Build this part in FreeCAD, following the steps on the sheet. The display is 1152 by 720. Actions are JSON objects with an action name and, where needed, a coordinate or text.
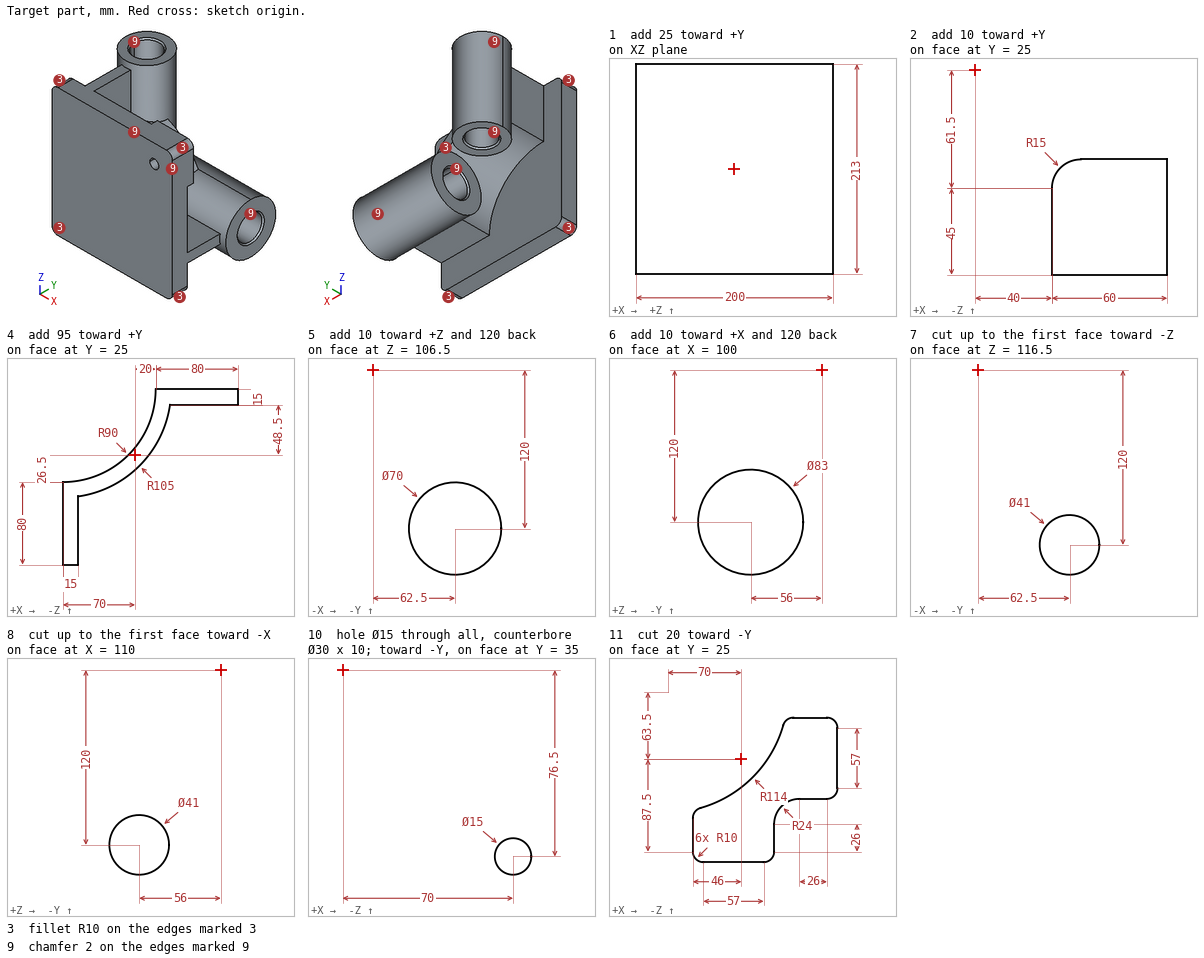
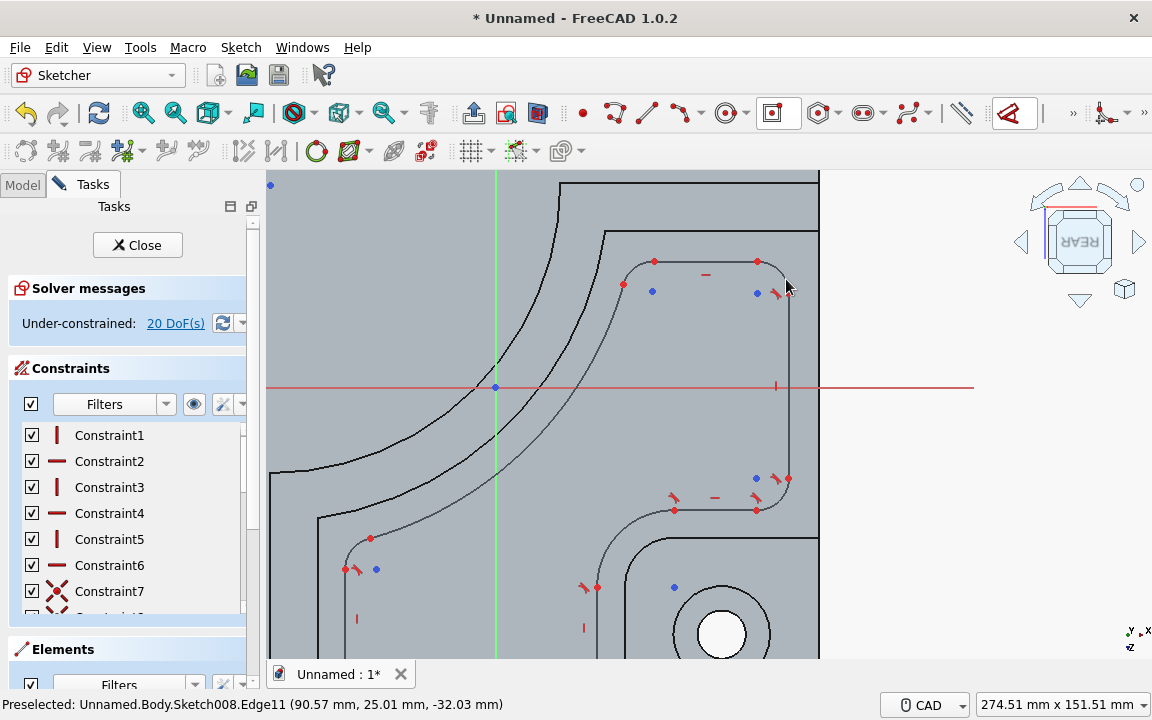
{"action": "left_click", "coordinate": [727, 262]}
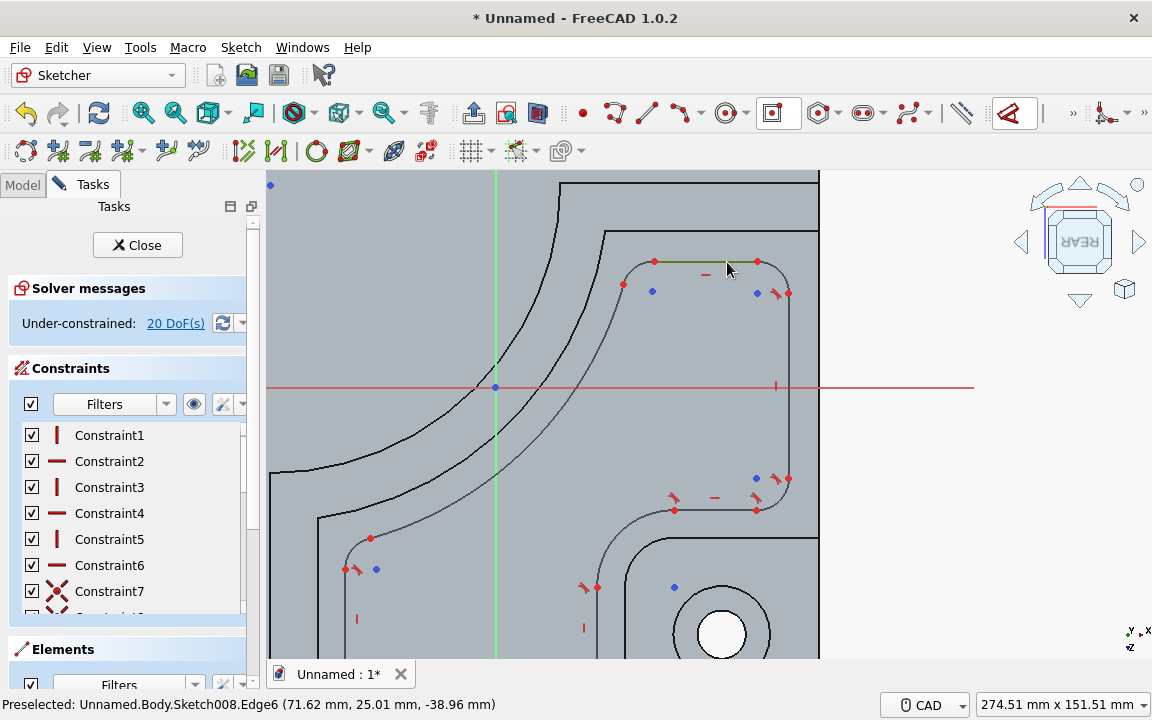
{"action": "left_click", "coordinate": [786, 279]}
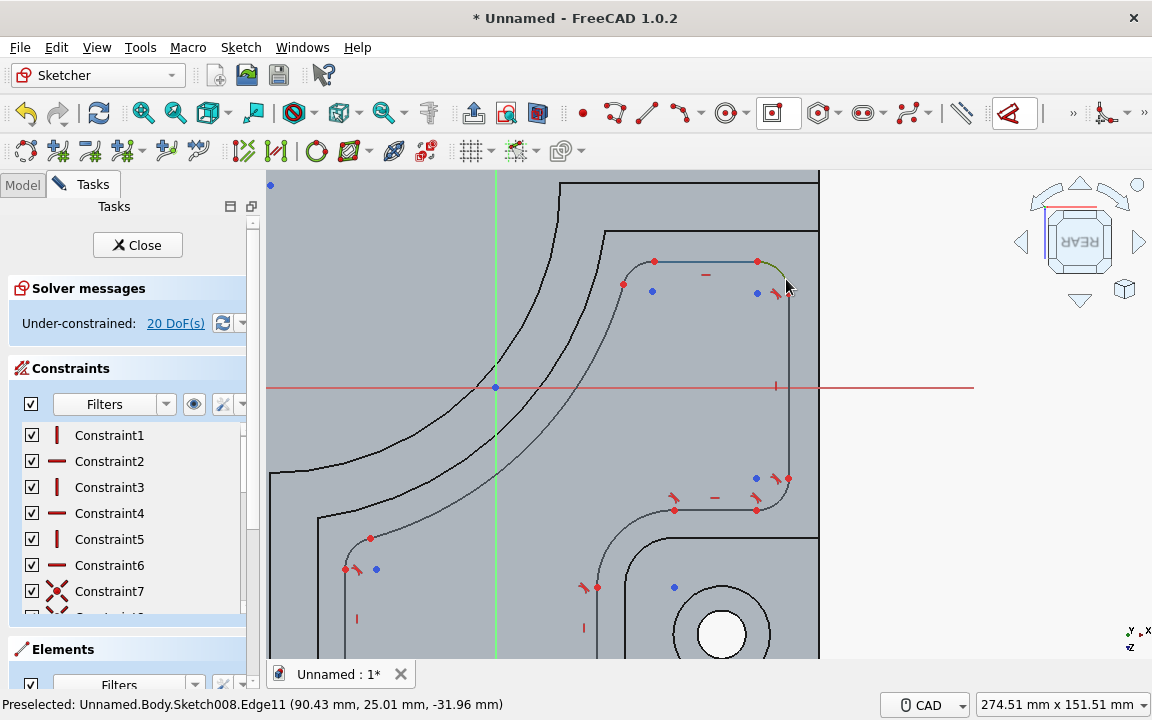
{"action": "key", "text": "t"}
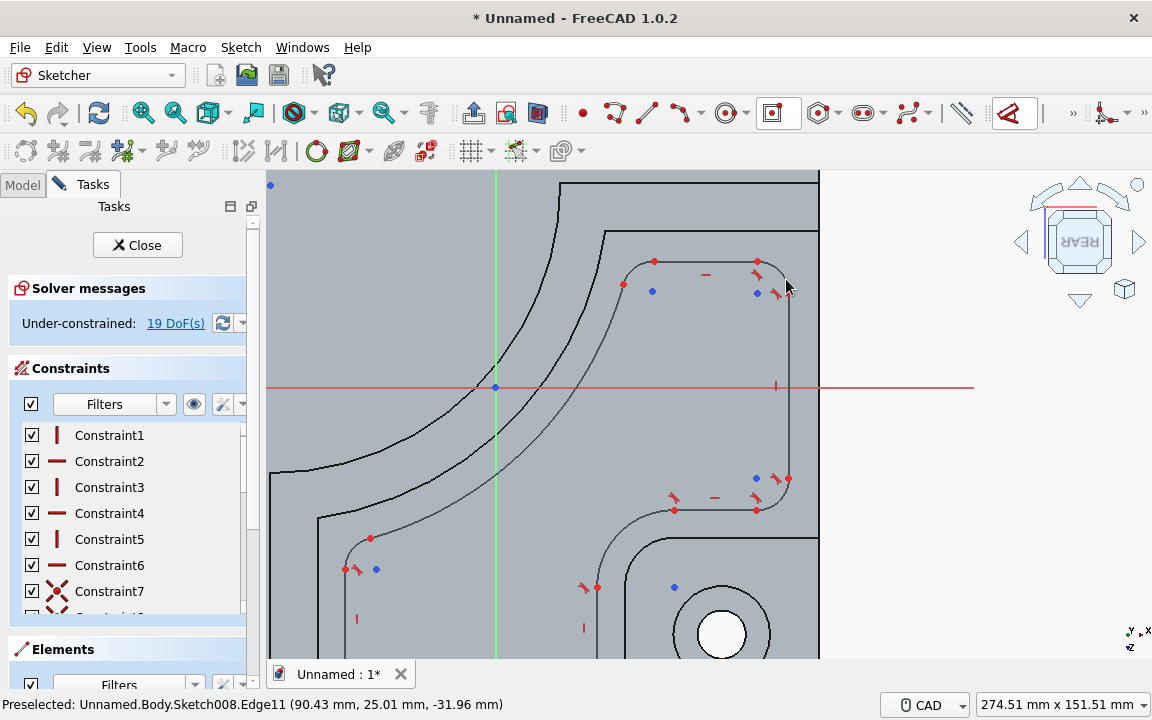
{"action": "left_click", "coordinate": [727, 262]}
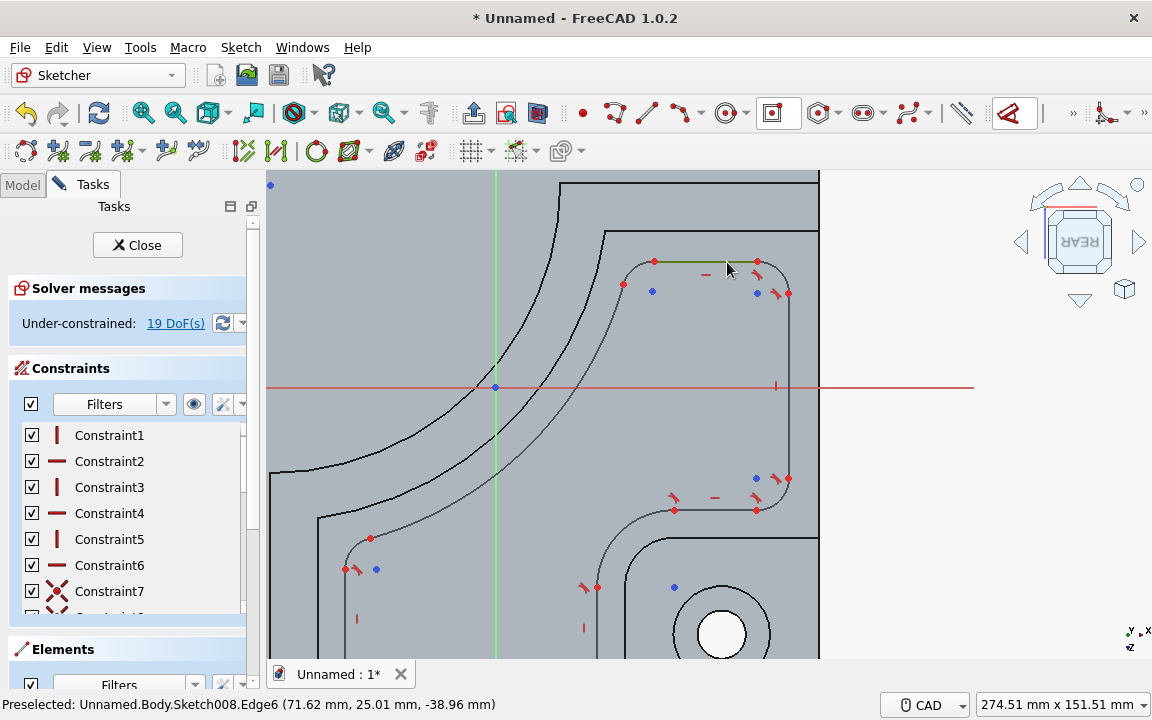
{"action": "left_click", "coordinate": [642, 264]}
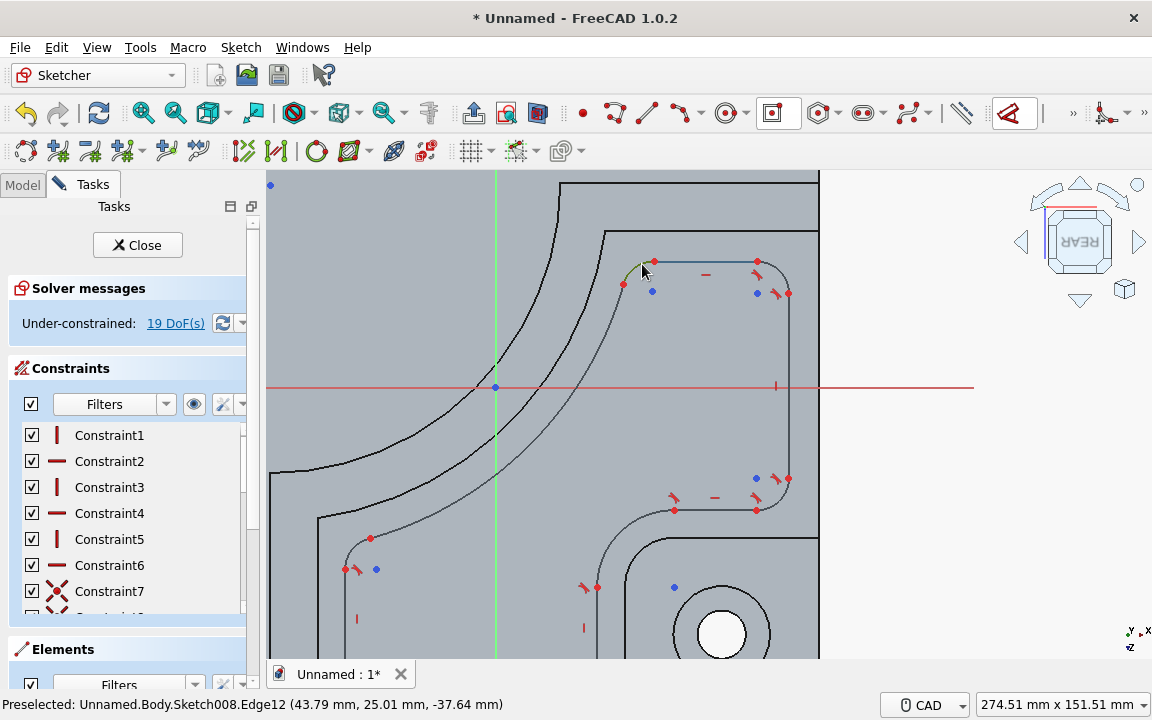
{"action": "key", "text": "t"}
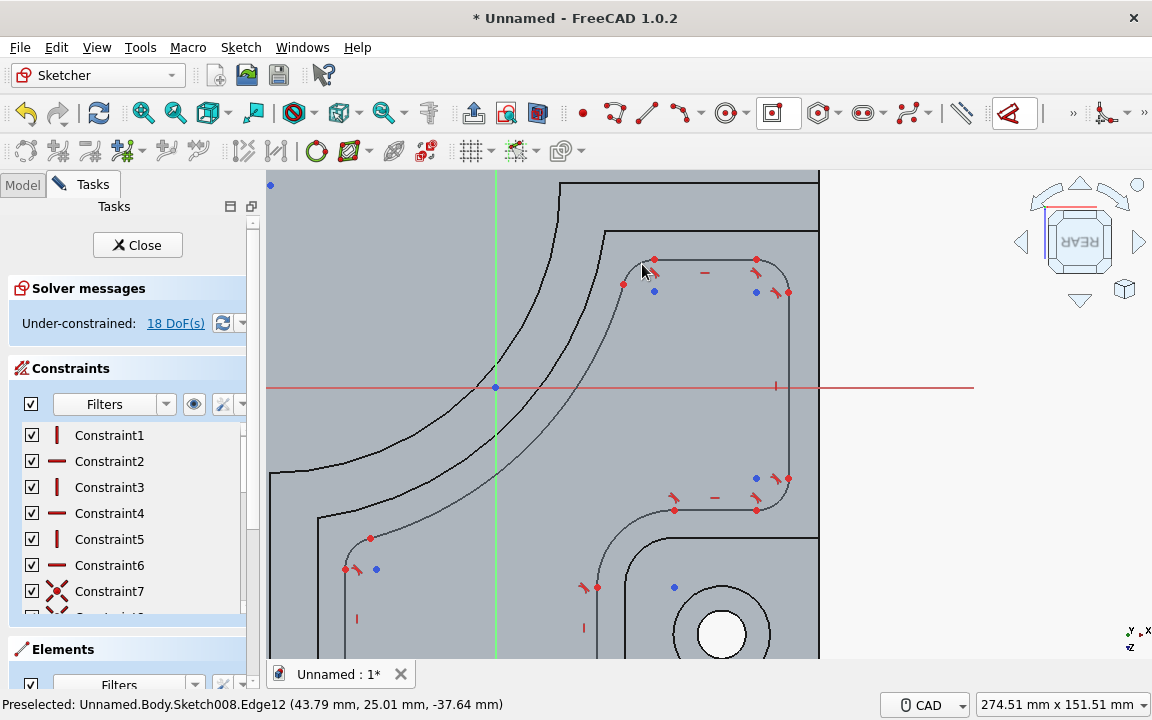
{"action": "left_click", "coordinate": [642, 262]}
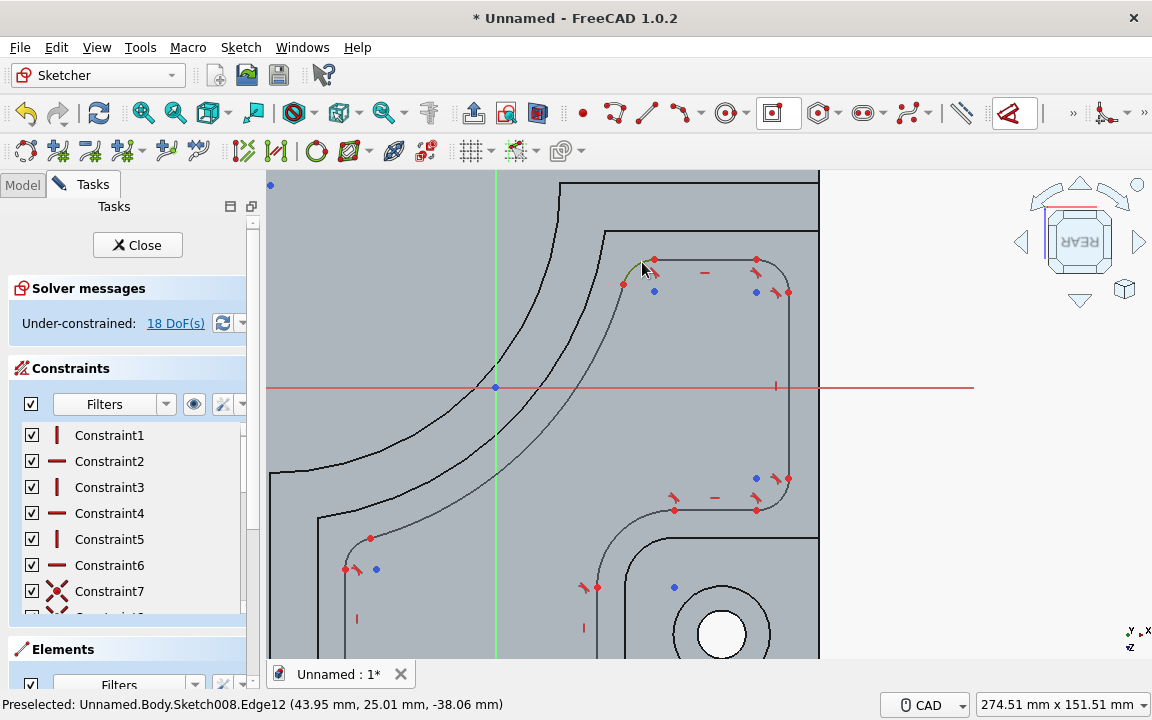
{"action": "left_click", "coordinate": [472, 492]}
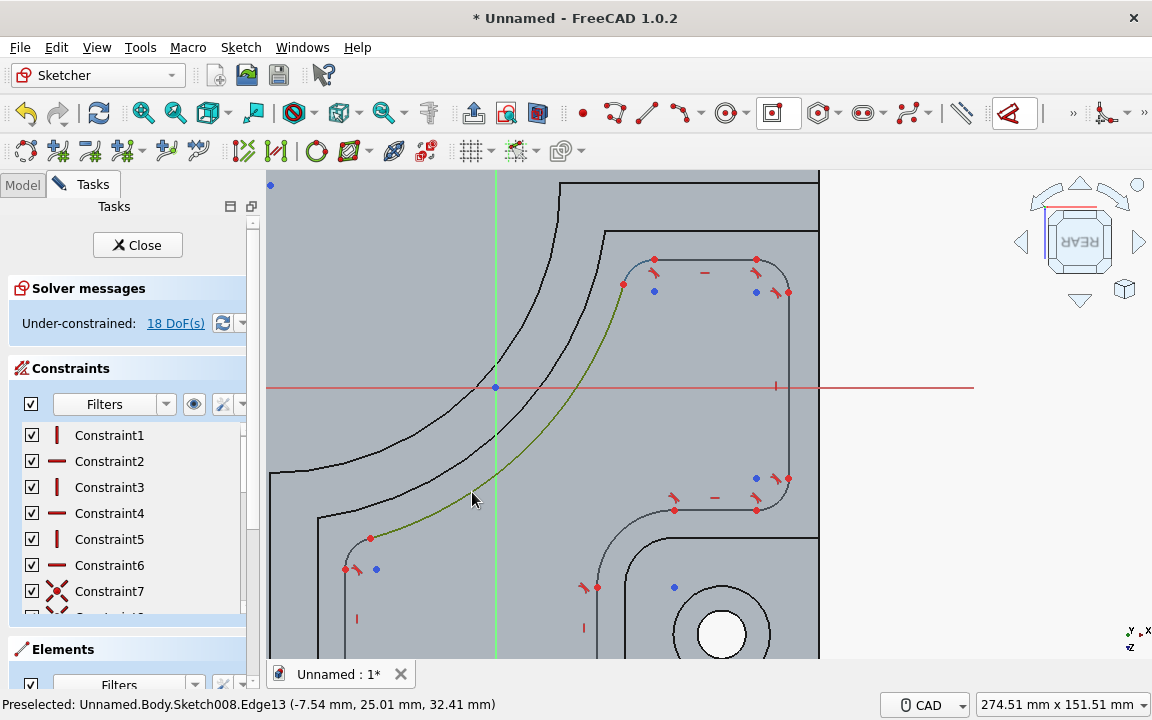
{"action": "key", "text": "t"}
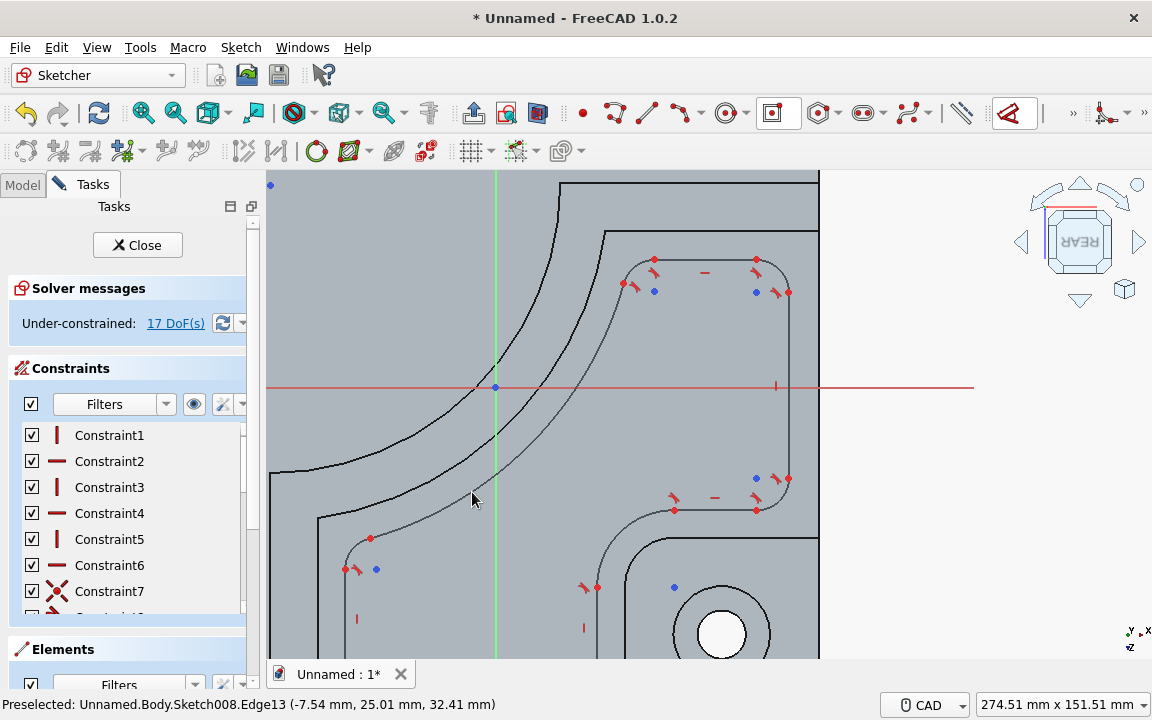
{"action": "left_click", "coordinate": [473, 492]}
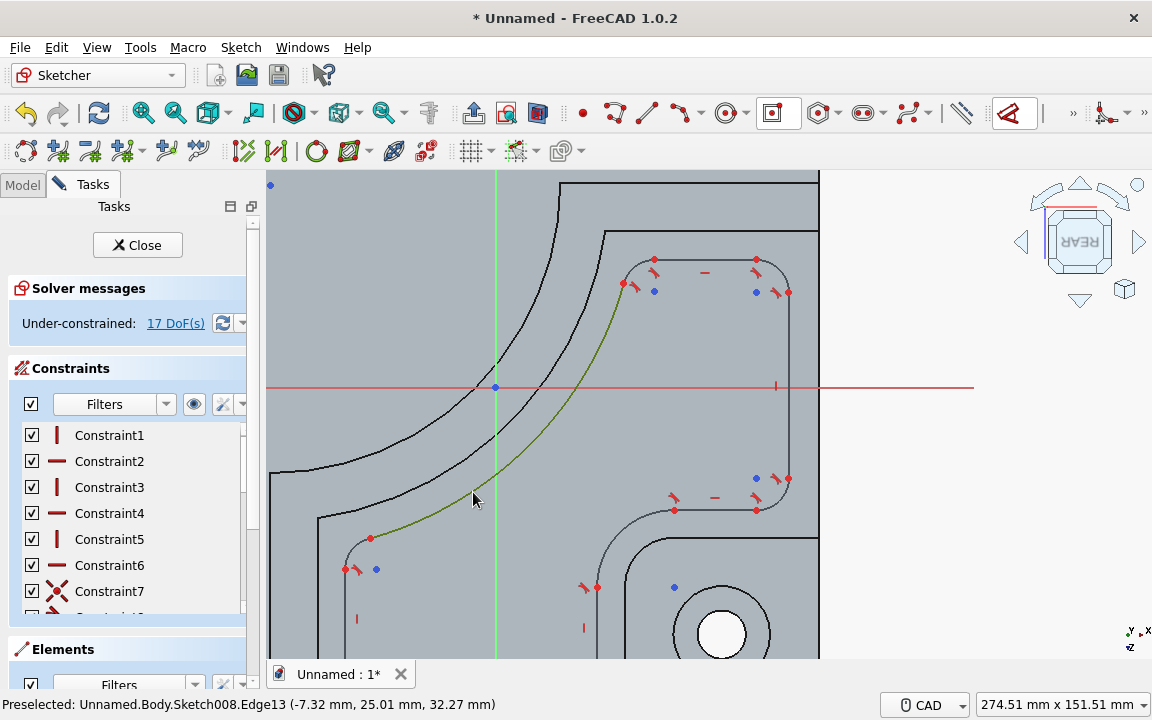
{"action": "left_click", "coordinate": [359, 543]}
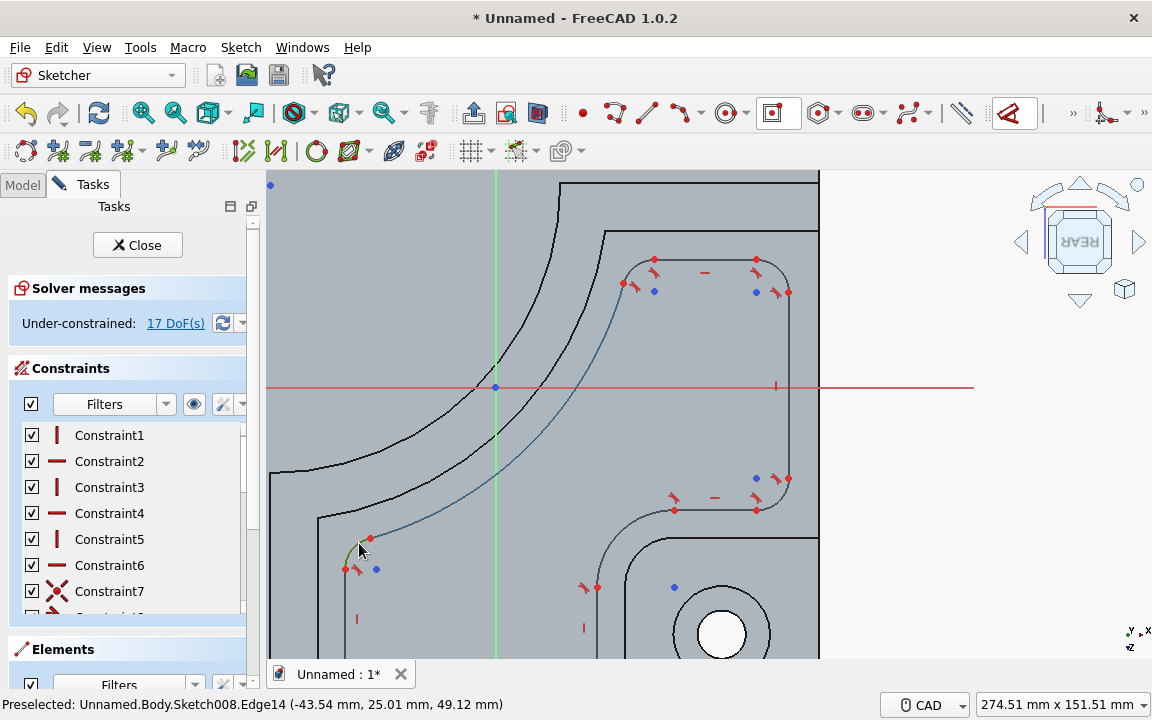
{"action": "key", "text": "t"}